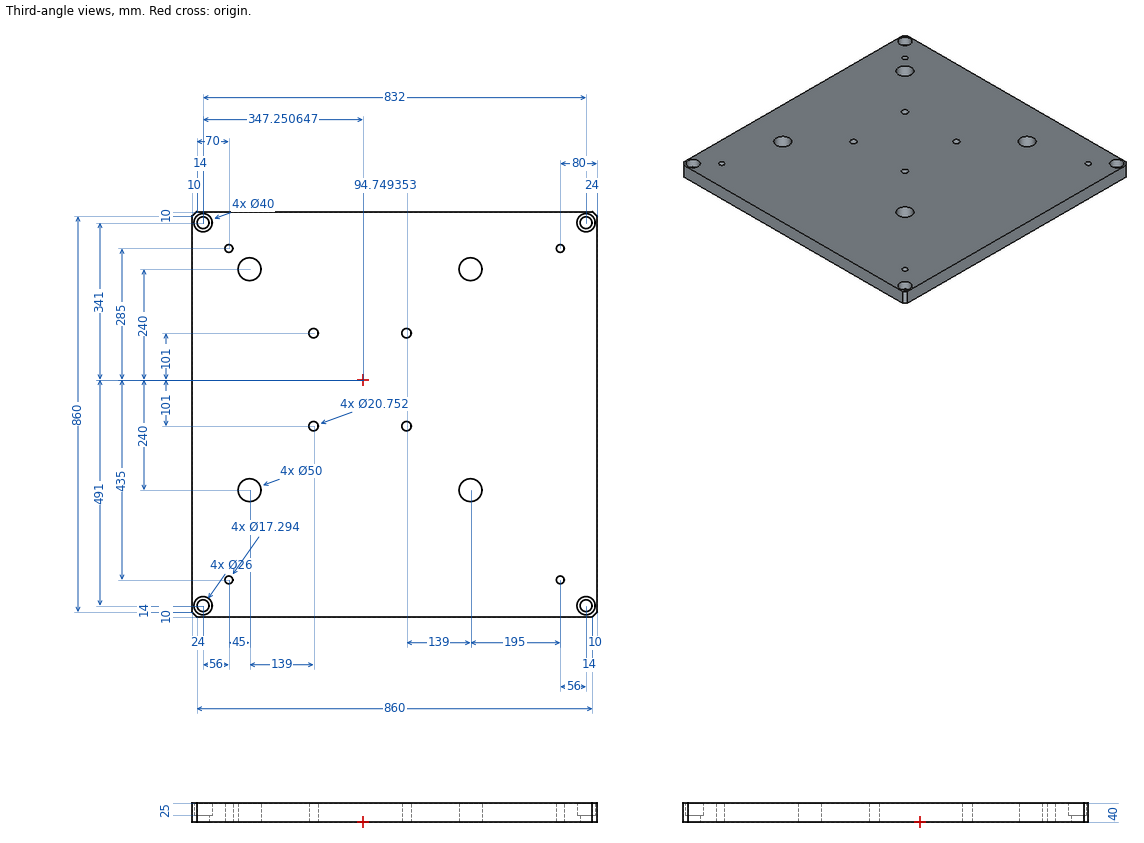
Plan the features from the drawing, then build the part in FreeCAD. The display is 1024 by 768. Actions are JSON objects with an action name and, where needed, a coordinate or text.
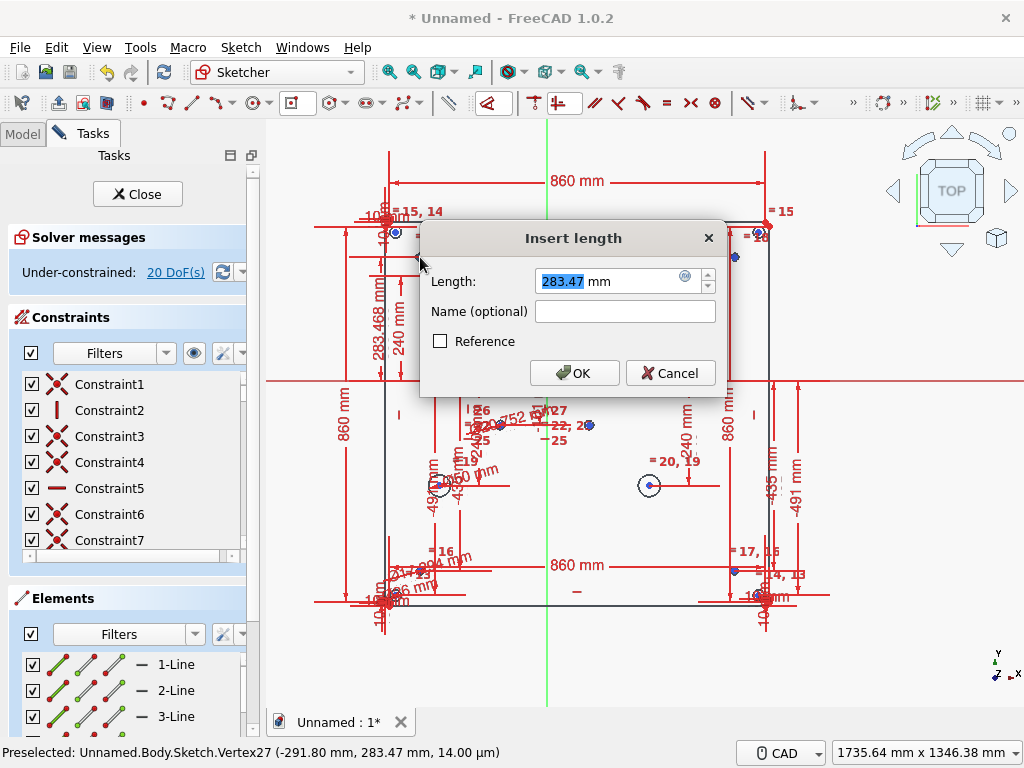
{"action": "type", "text": "285"}
{"action": "key", "text": "Return"}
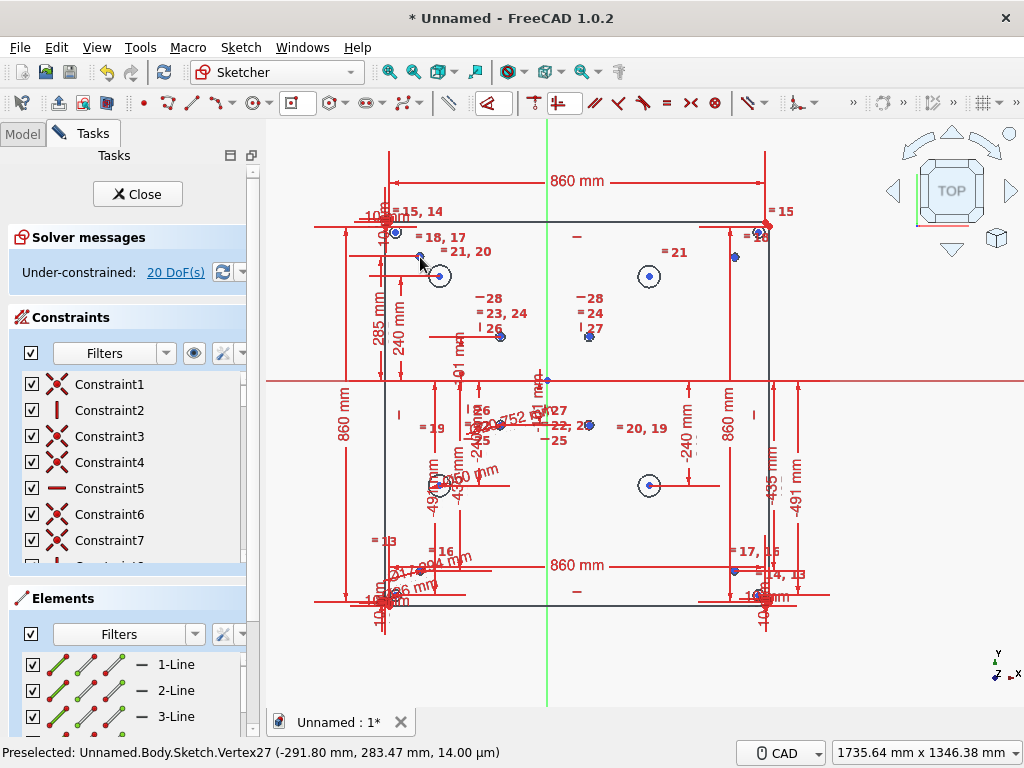
{"action": "left_click", "coordinate": [396, 232]}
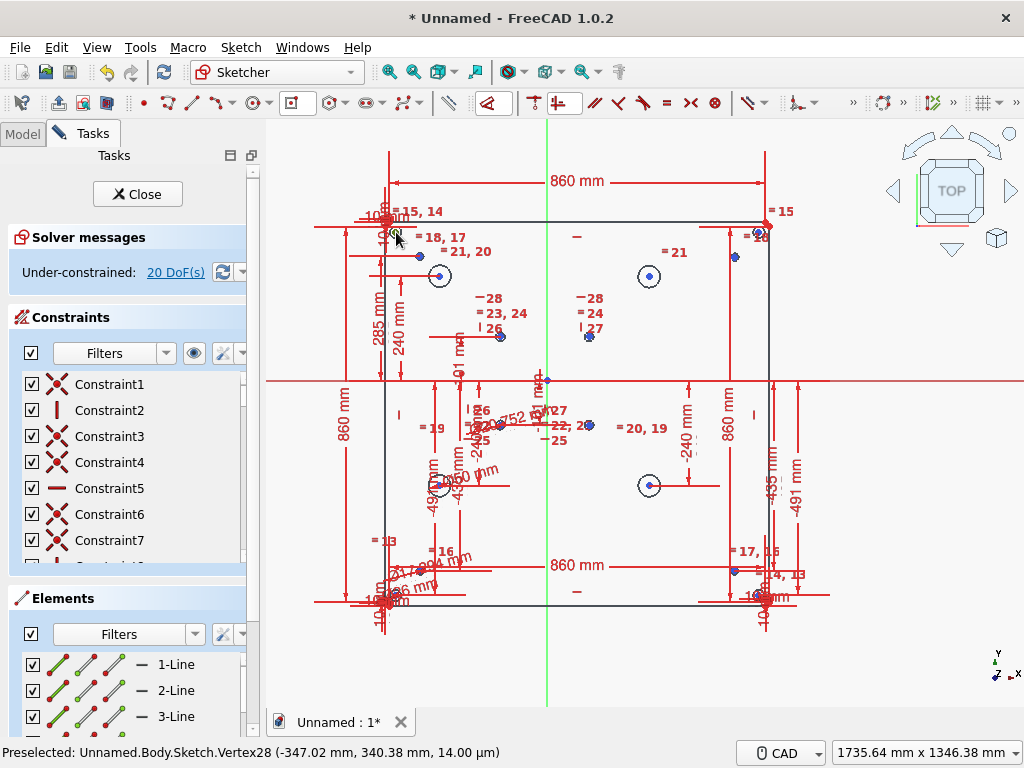
{"action": "left_click", "coordinate": [506, 104]}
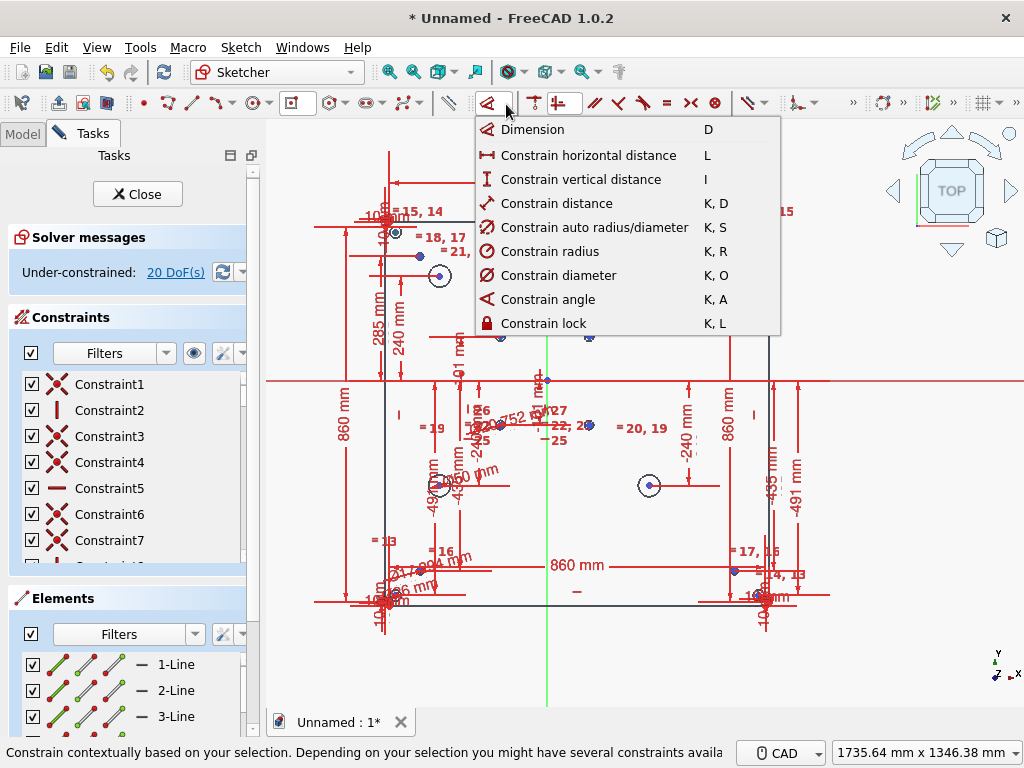
{"action": "left_click", "coordinate": [628, 179]}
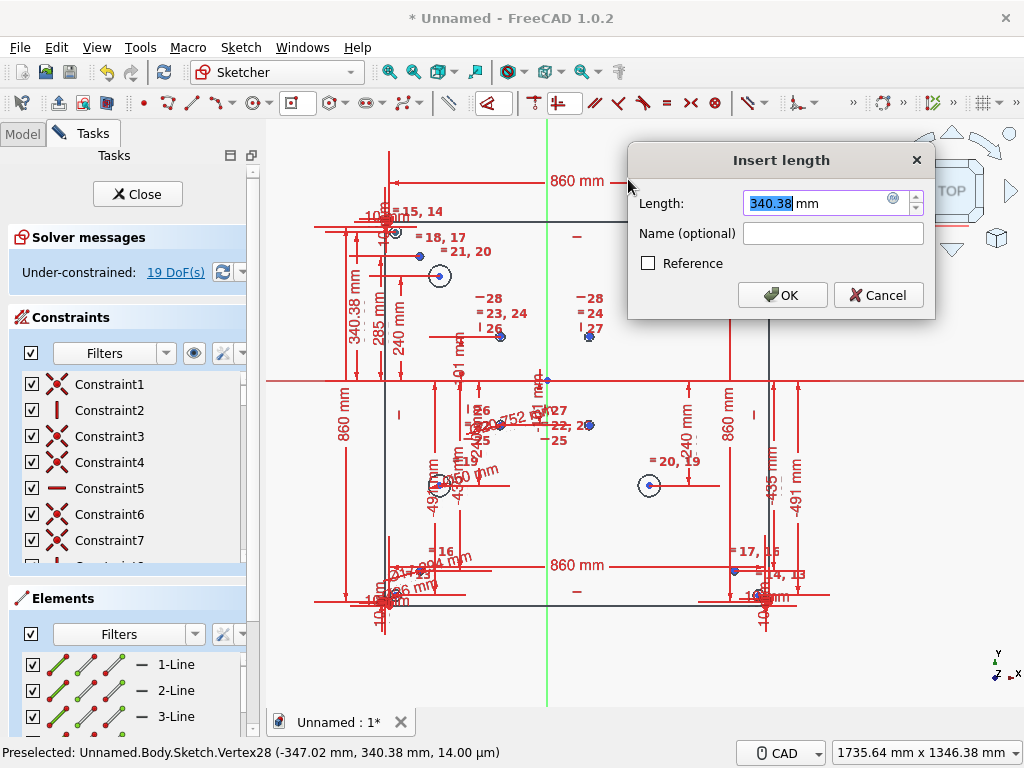
{"action": "type", "text": "341"}
{"action": "key", "text": "Return"}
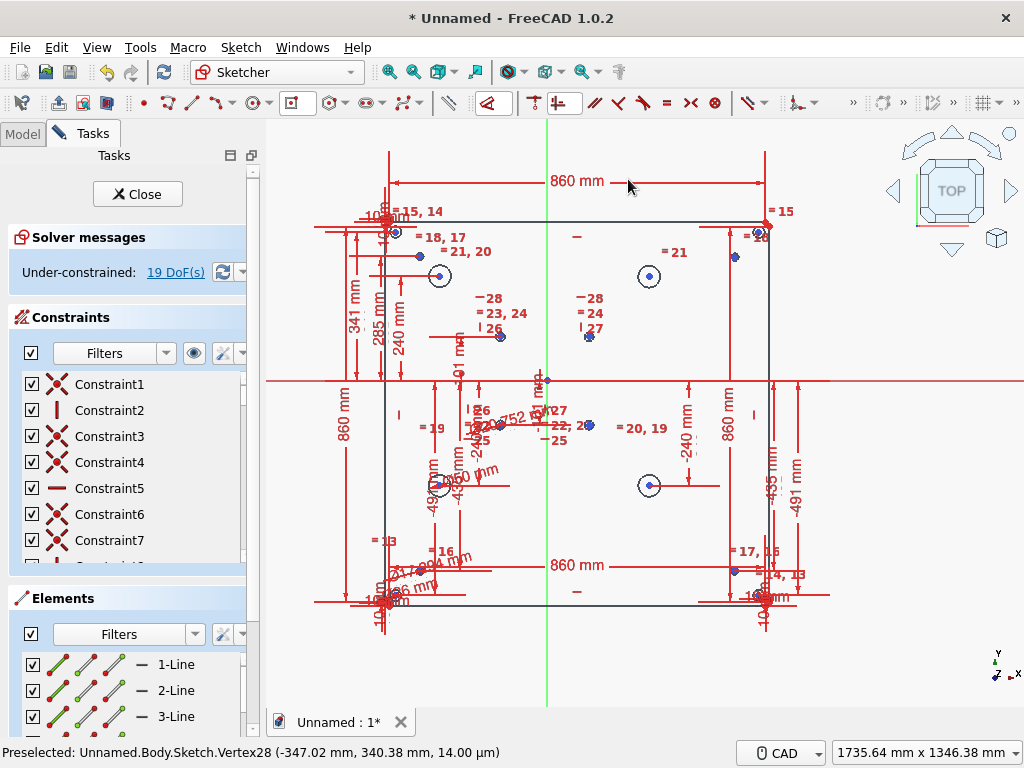
{"action": "left_click", "coordinate": [649, 277]}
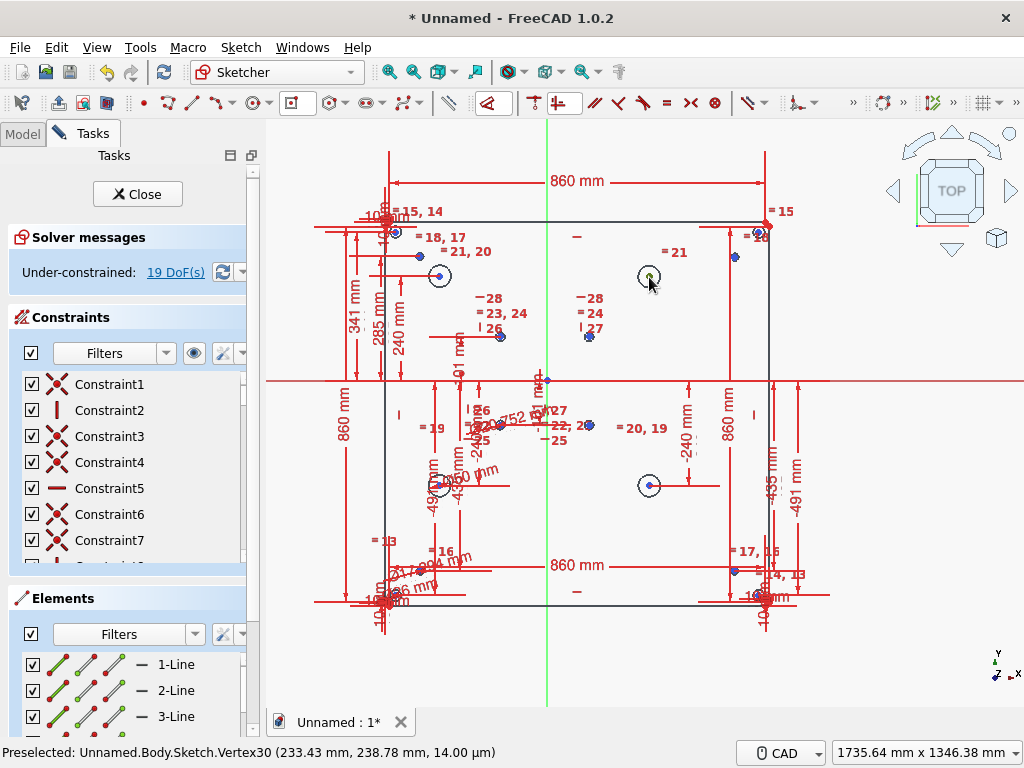
{"action": "left_click", "coordinate": [506, 104]}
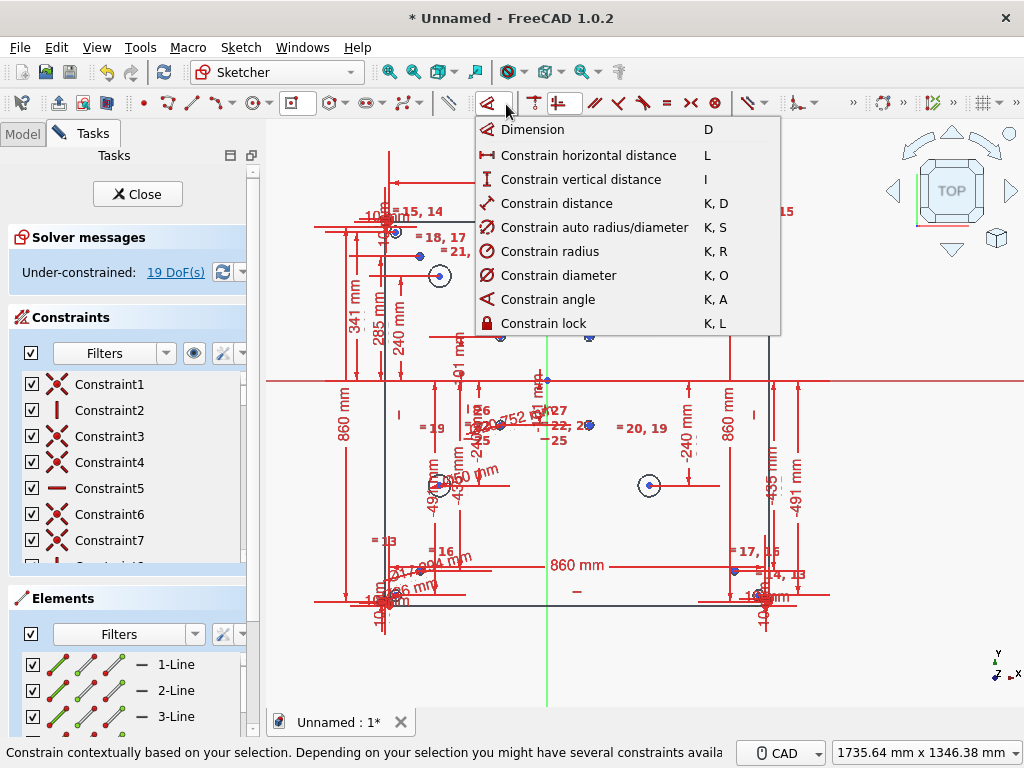
{"action": "left_click", "coordinate": [628, 179]}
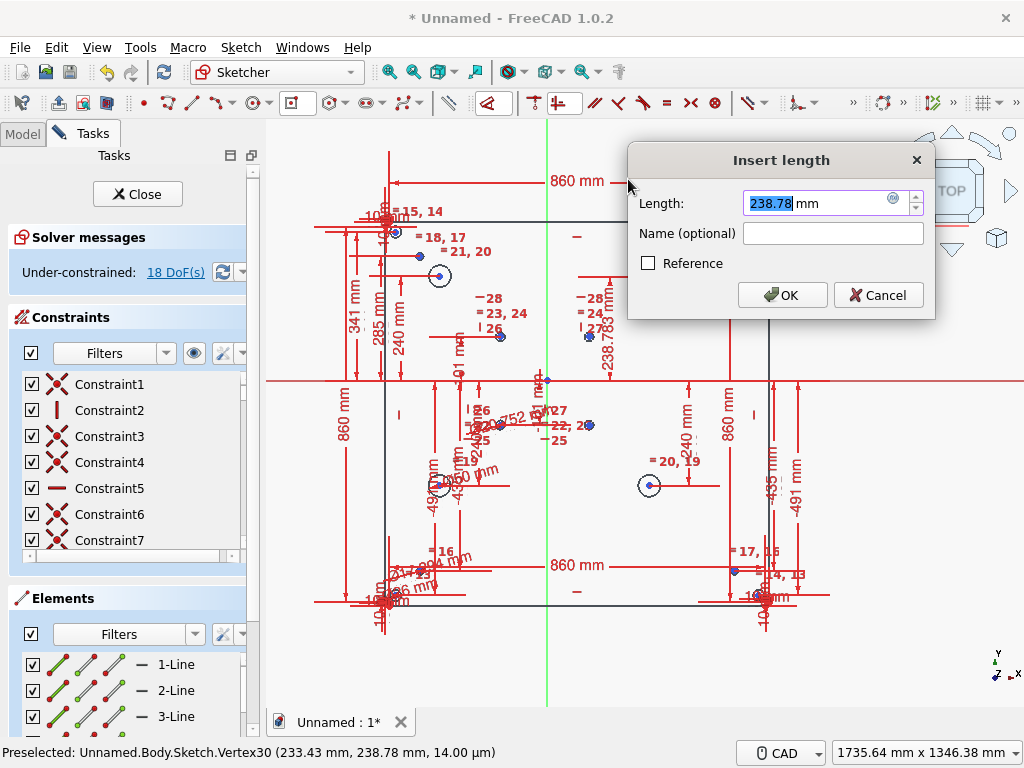
{"action": "type", "text": "240"}
{"action": "key", "text": "Return"}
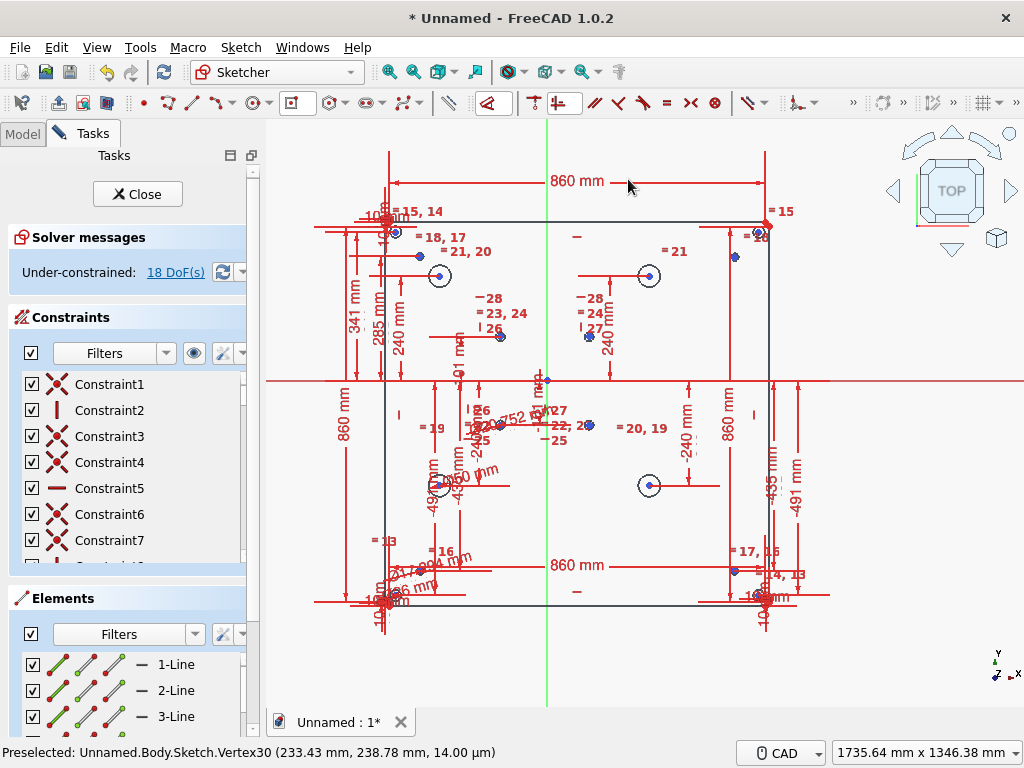
{"action": "left_click", "coordinate": [735, 257]}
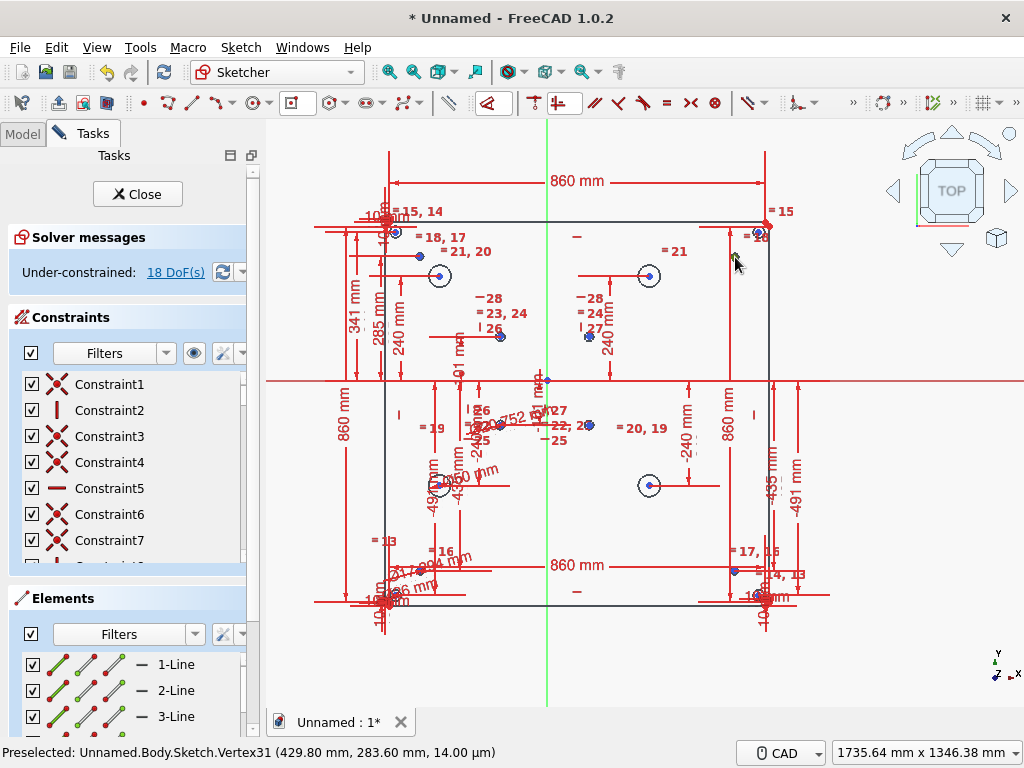
{"action": "key", "text": "i"}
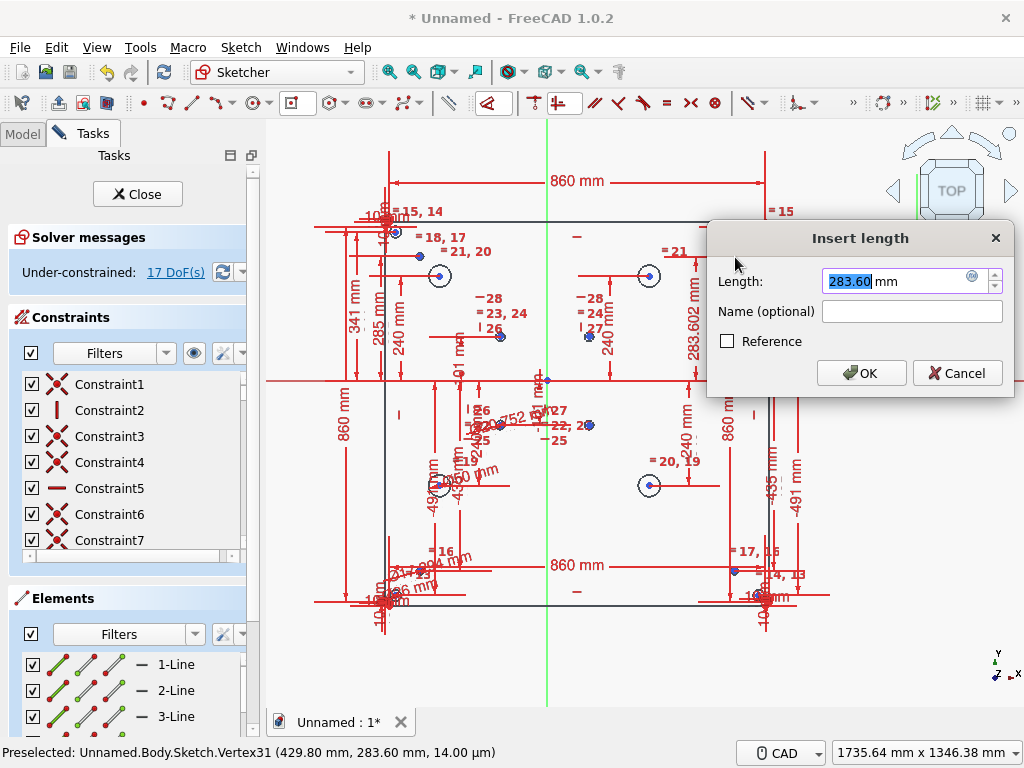
{"action": "type", "text": "285"}
{"action": "key", "text": "Return"}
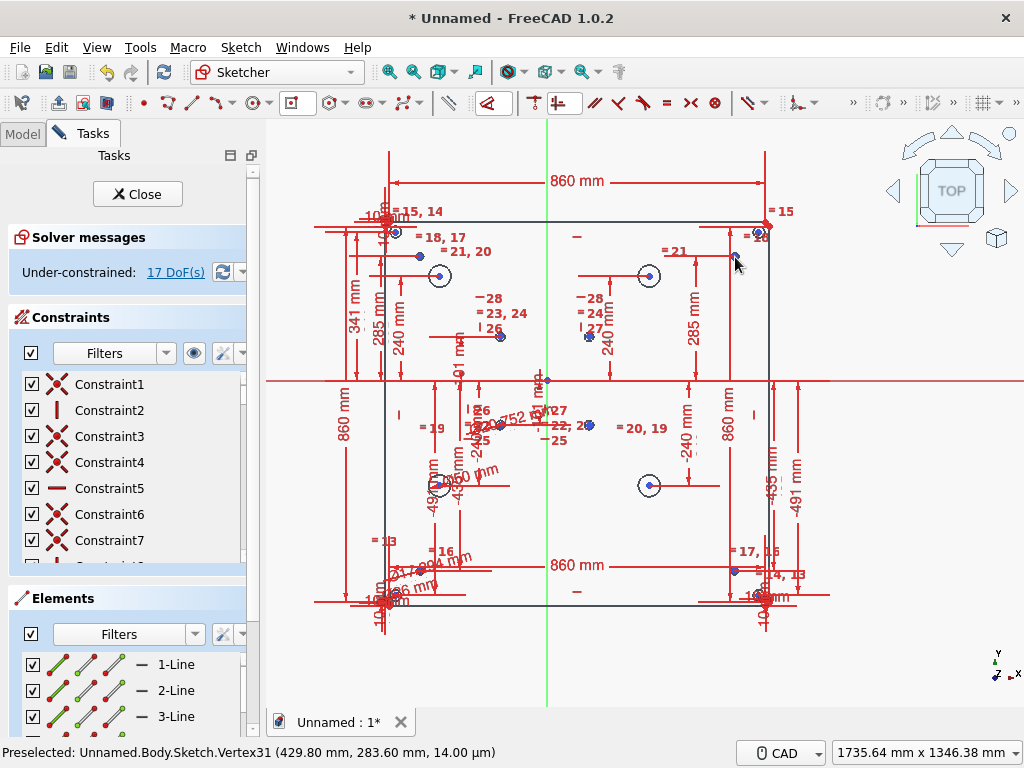
{"action": "scroll", "coordinate": [759, 232], "scroll_direction": "up", "scroll_amount": 4}